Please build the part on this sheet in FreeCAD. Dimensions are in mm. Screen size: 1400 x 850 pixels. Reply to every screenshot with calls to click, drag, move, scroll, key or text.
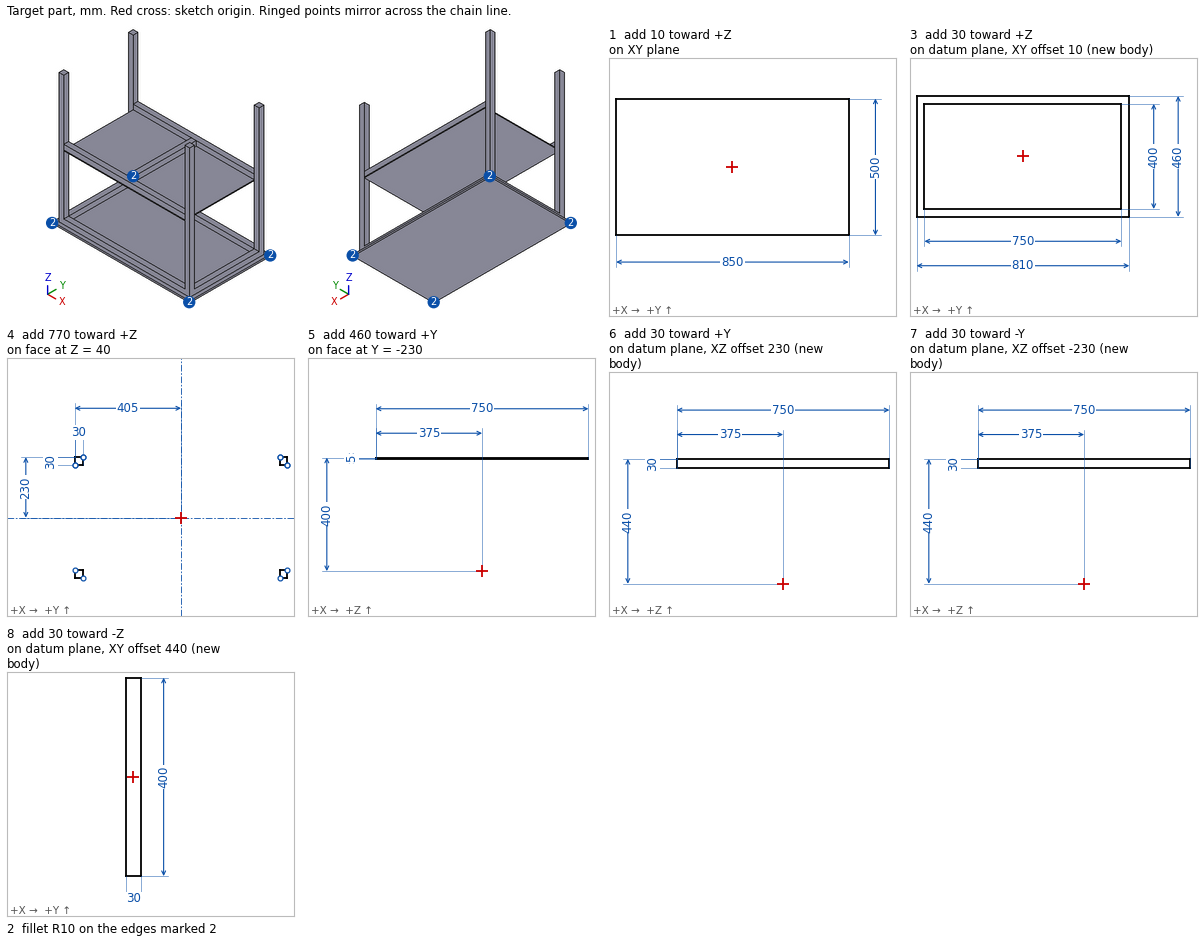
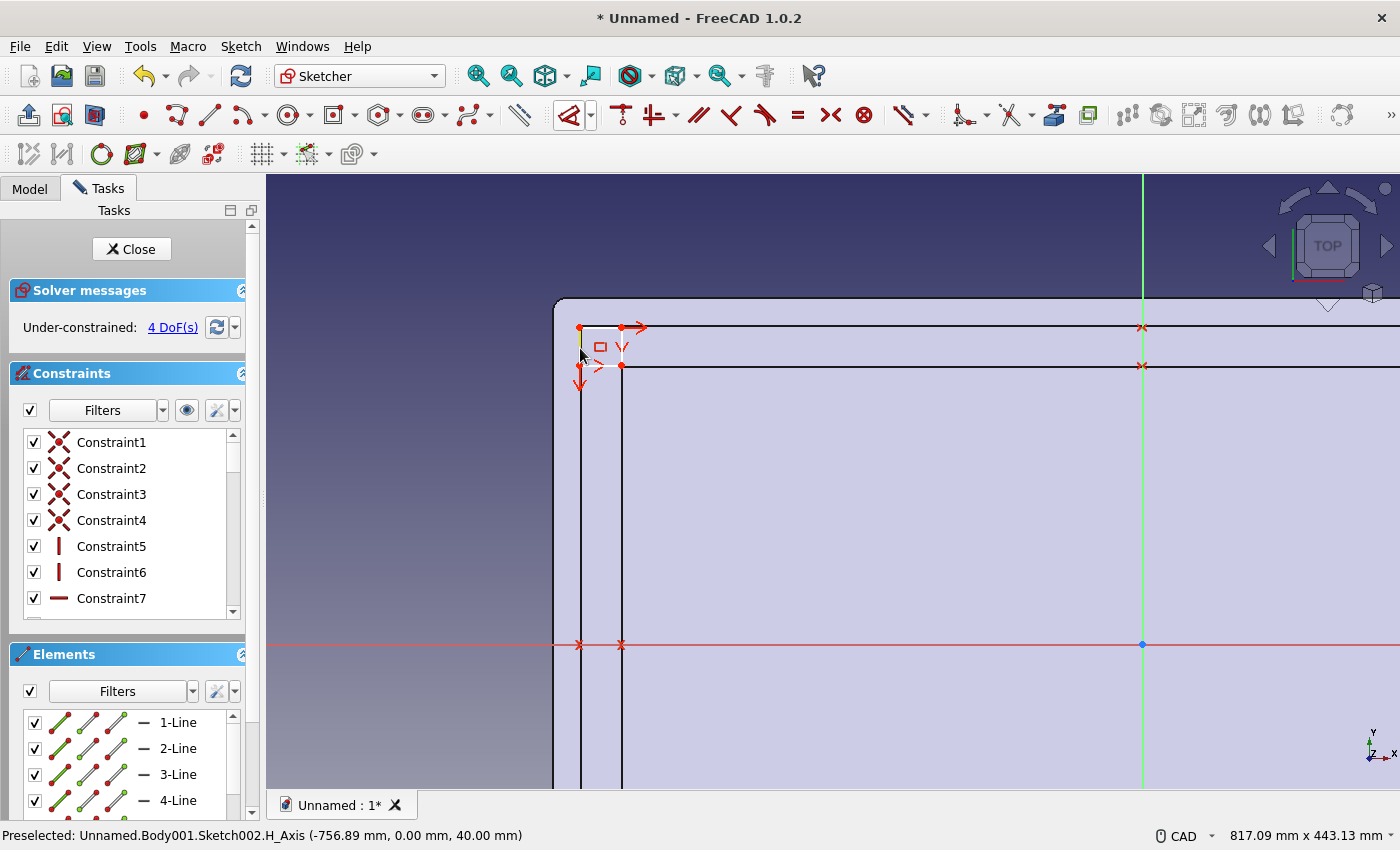
click(580, 347)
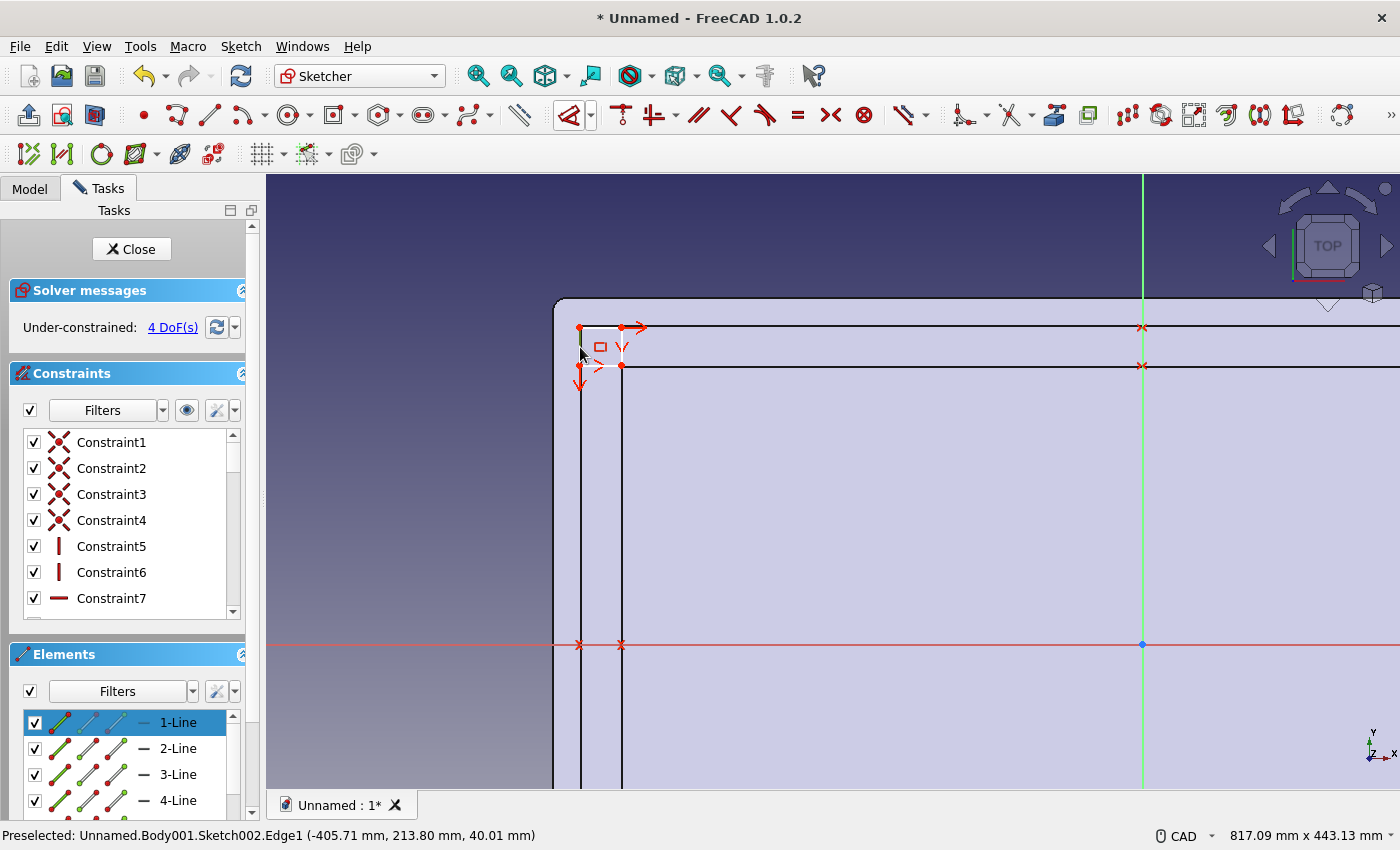
key(i)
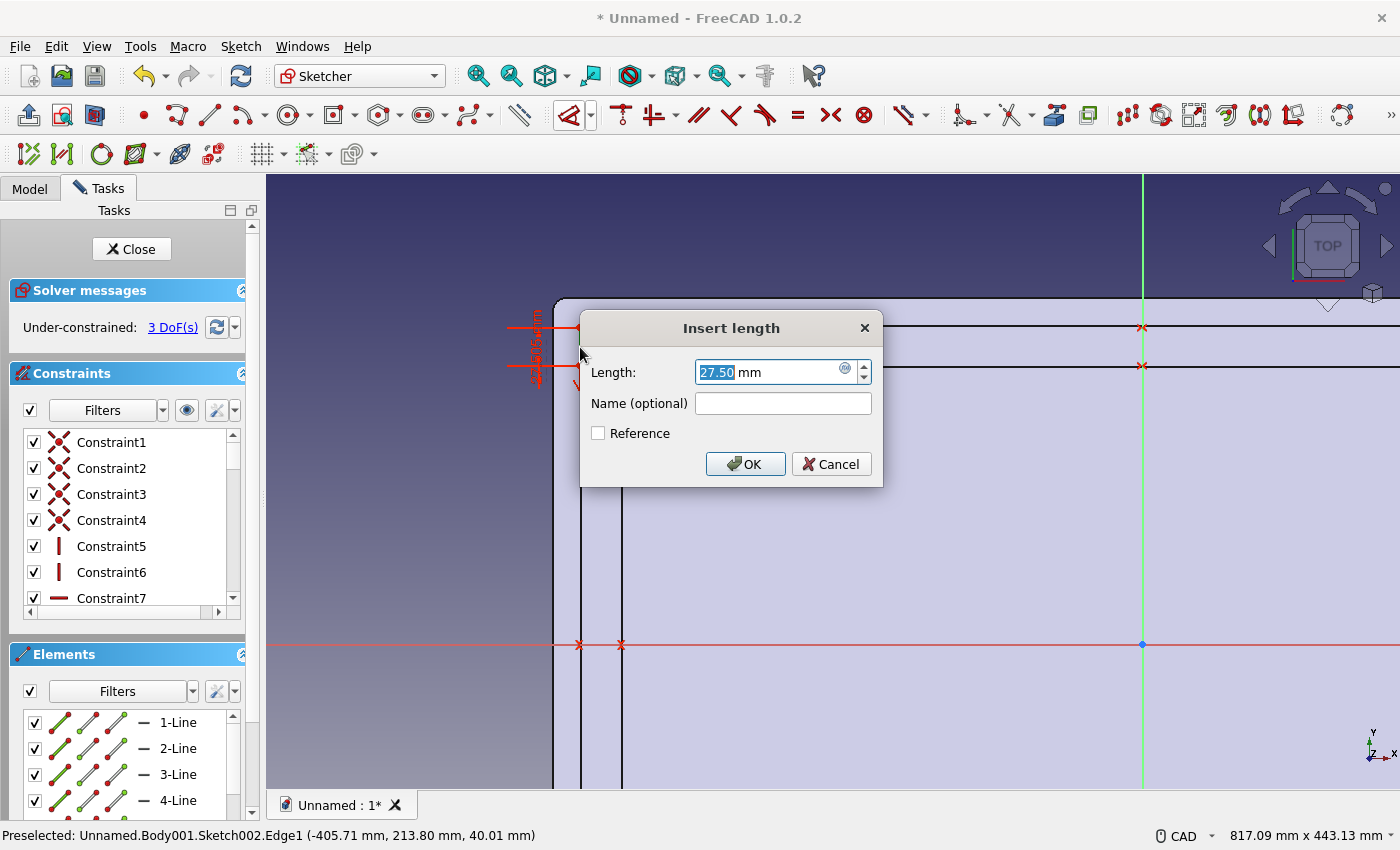
text(30)
key(Return)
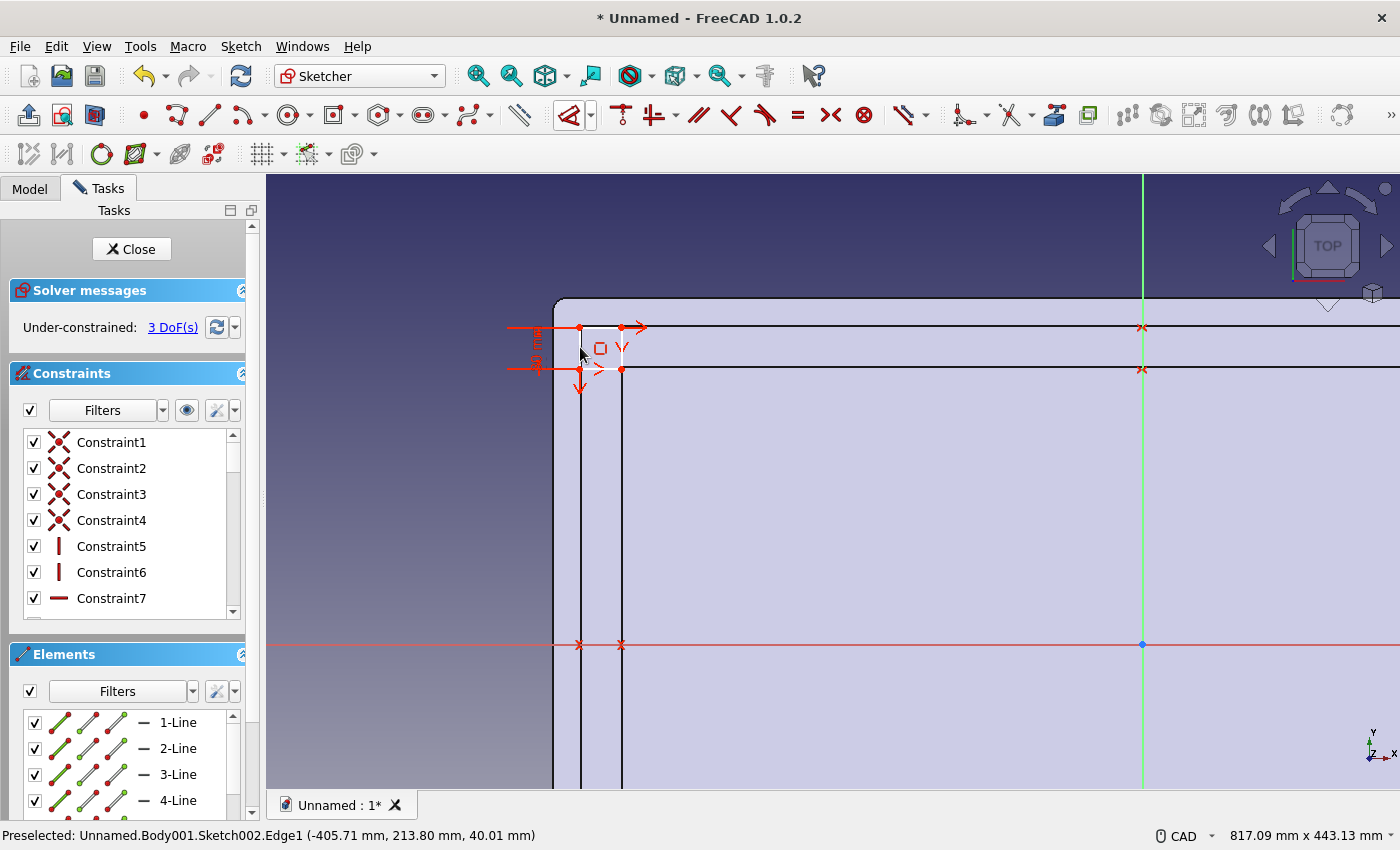
click(592, 369)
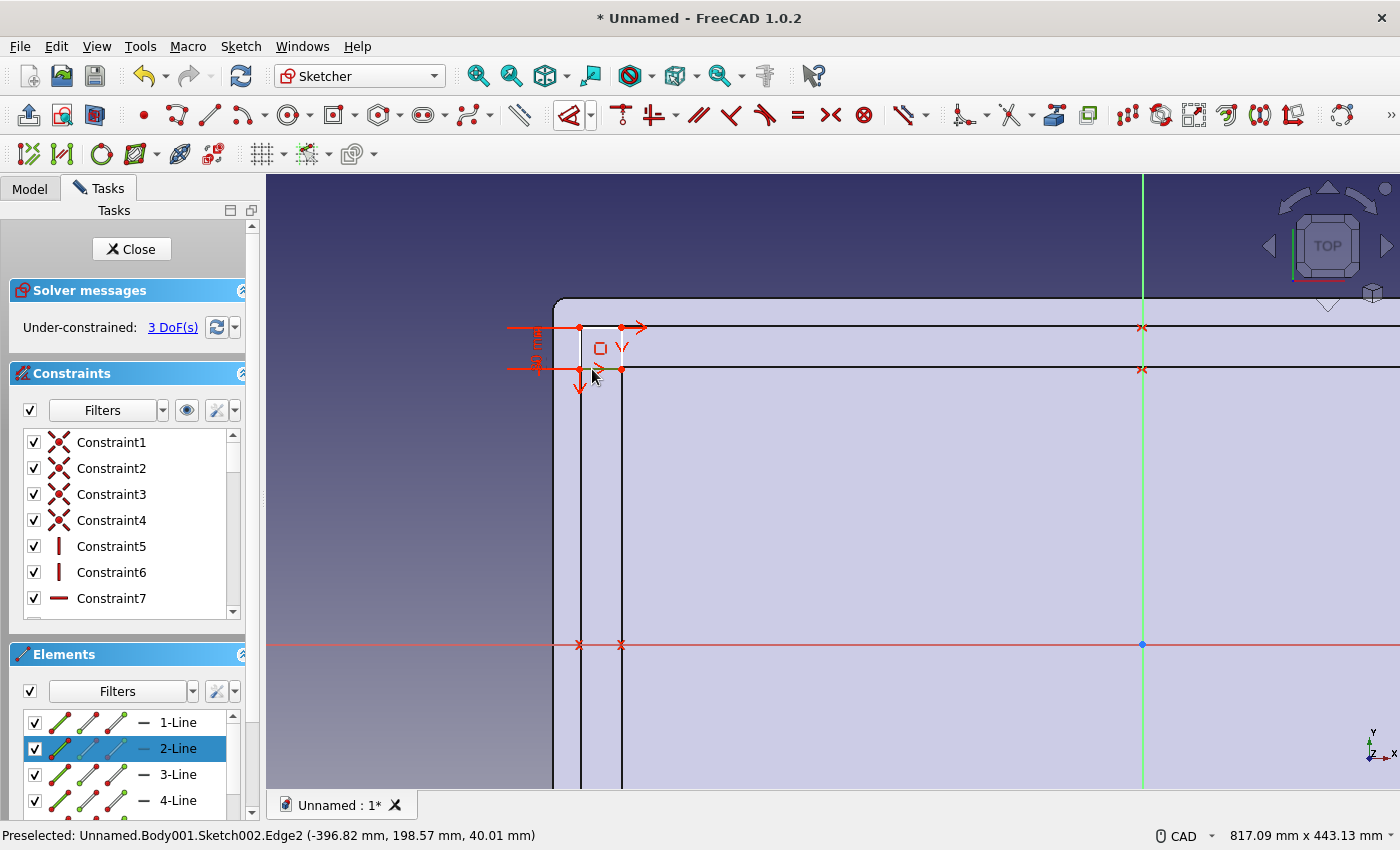
click(590, 116)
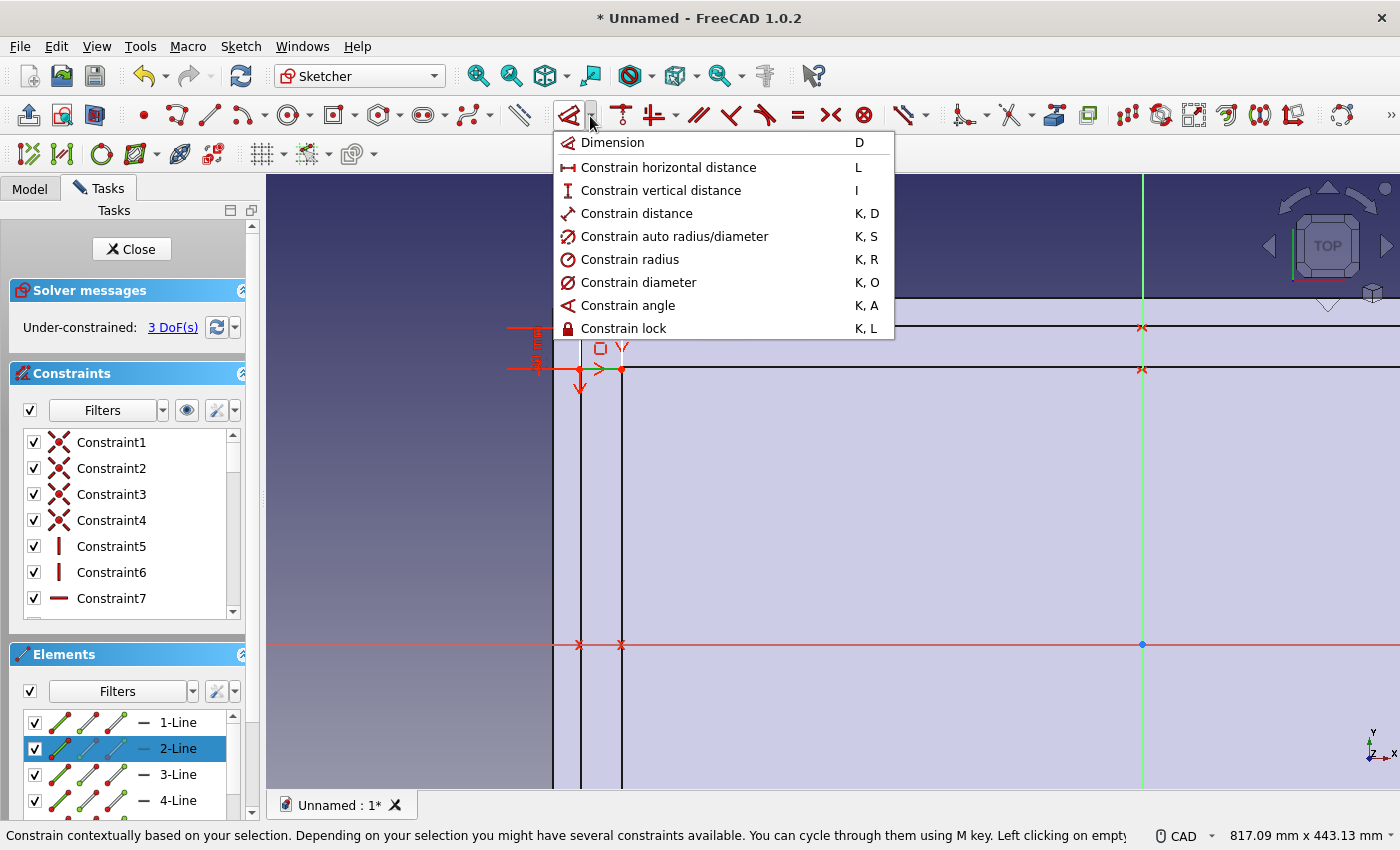
click(724, 168)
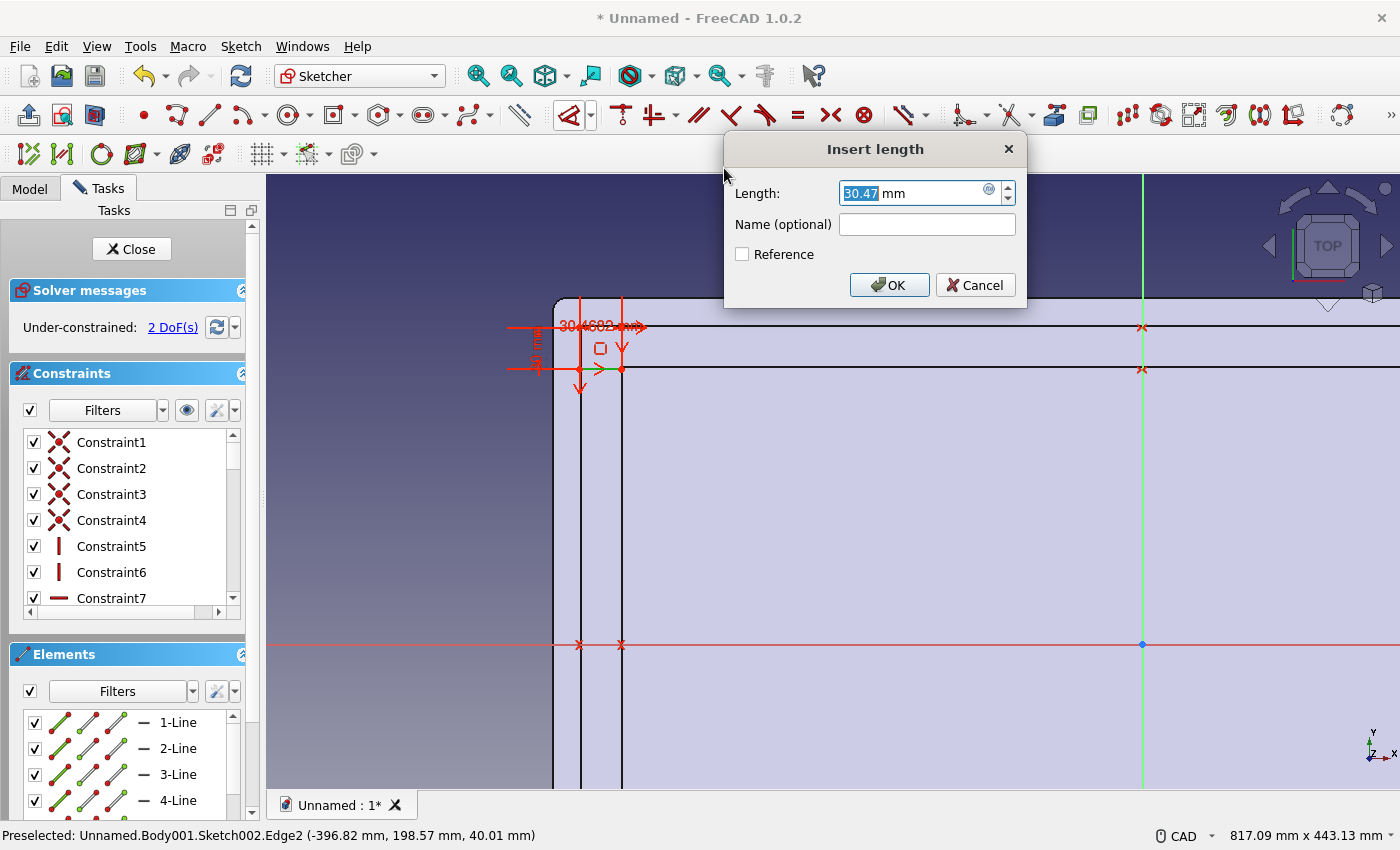
text(30)
key(Return)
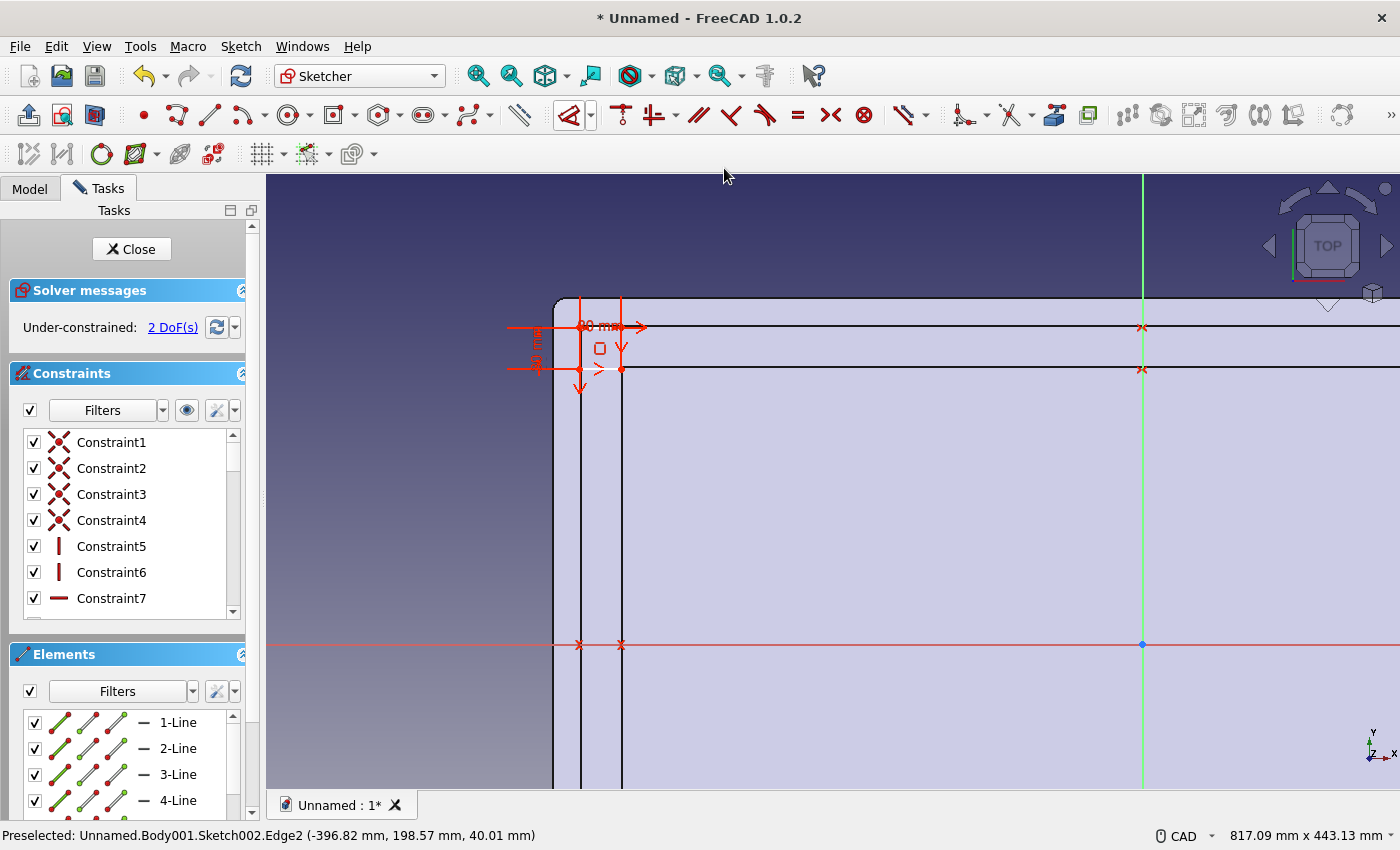
click(580, 328)